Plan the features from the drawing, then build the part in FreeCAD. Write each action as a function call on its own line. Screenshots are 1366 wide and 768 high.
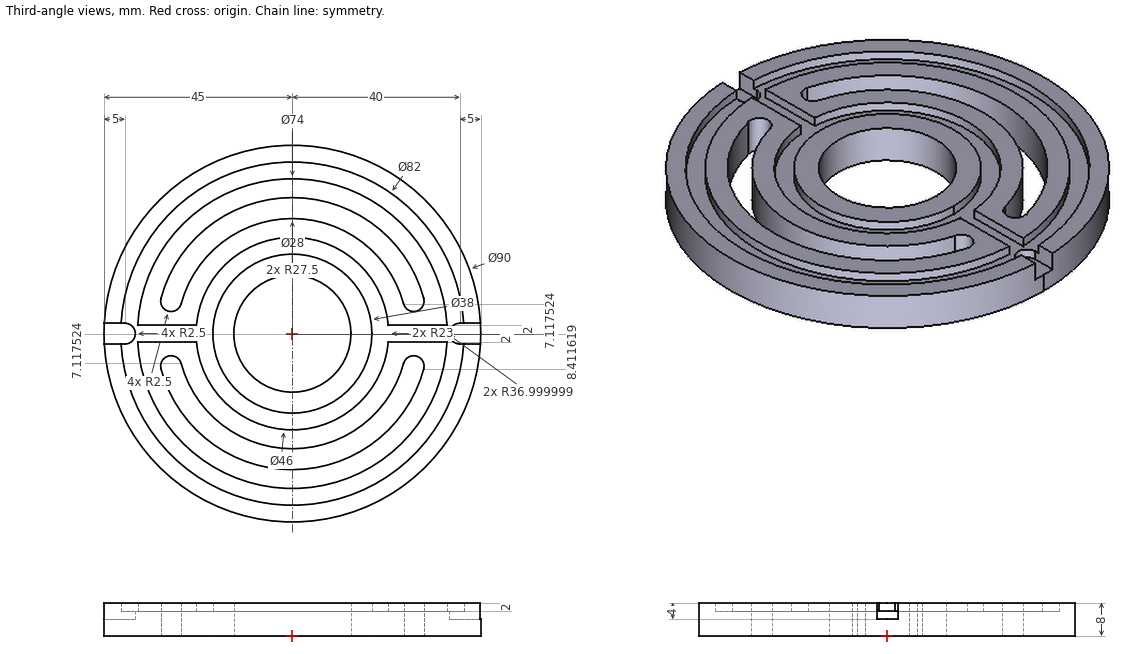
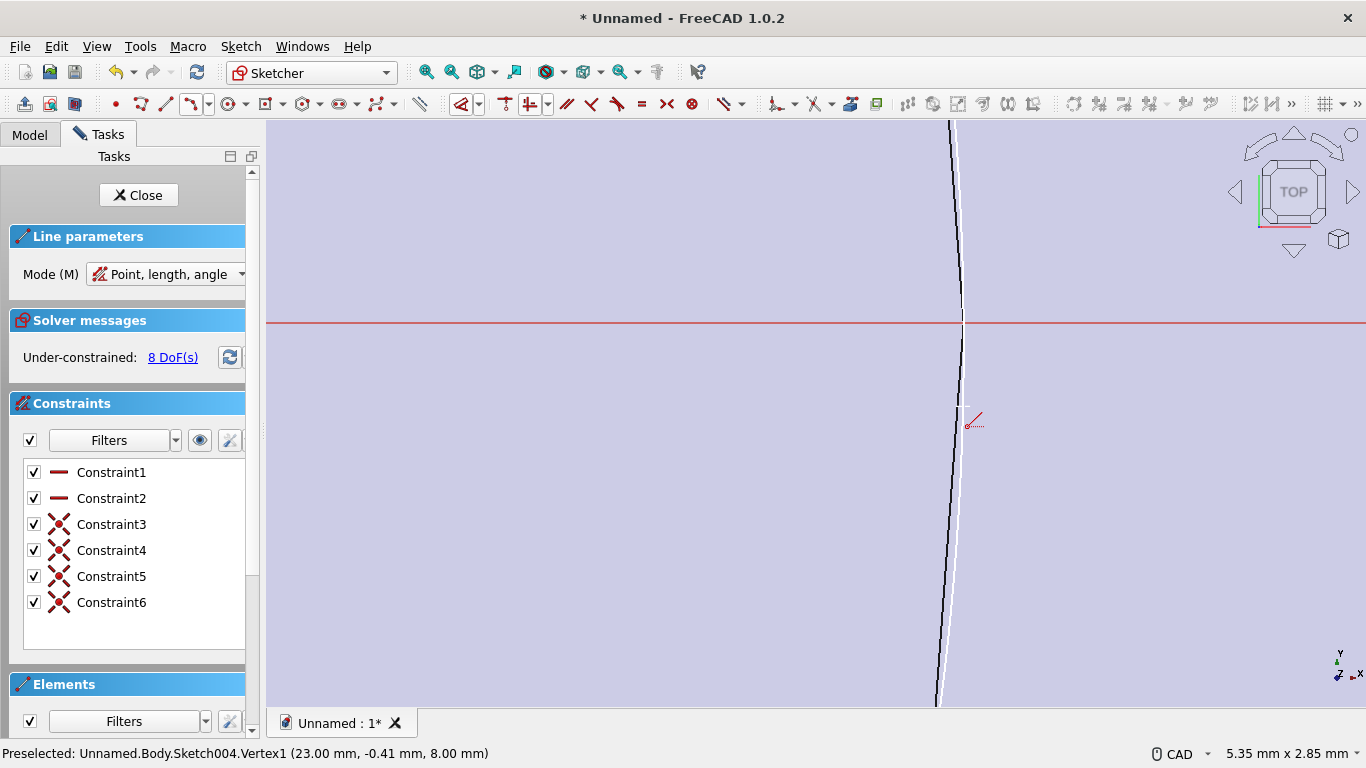
scroll(984, 418, down, 15)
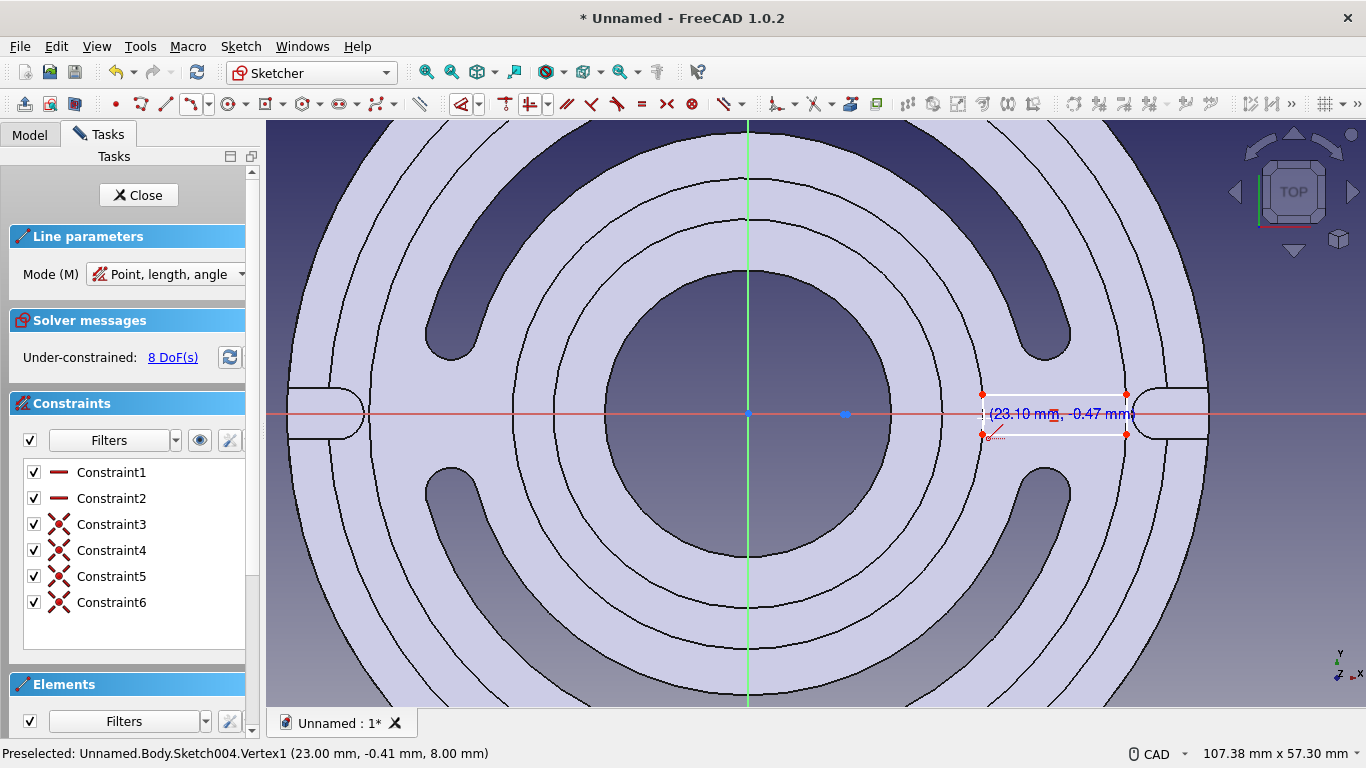
click(370, 434)
click(513, 434)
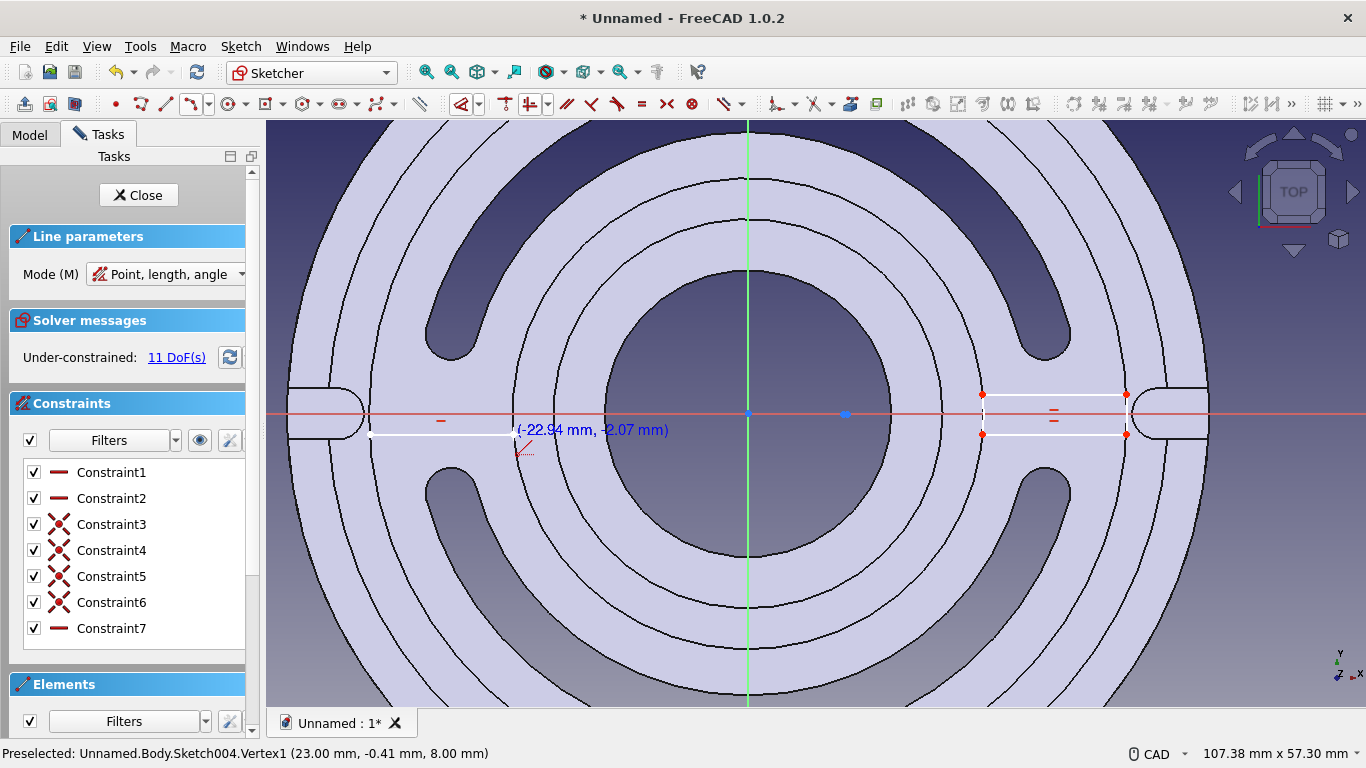
click(513, 393)
click(370, 393)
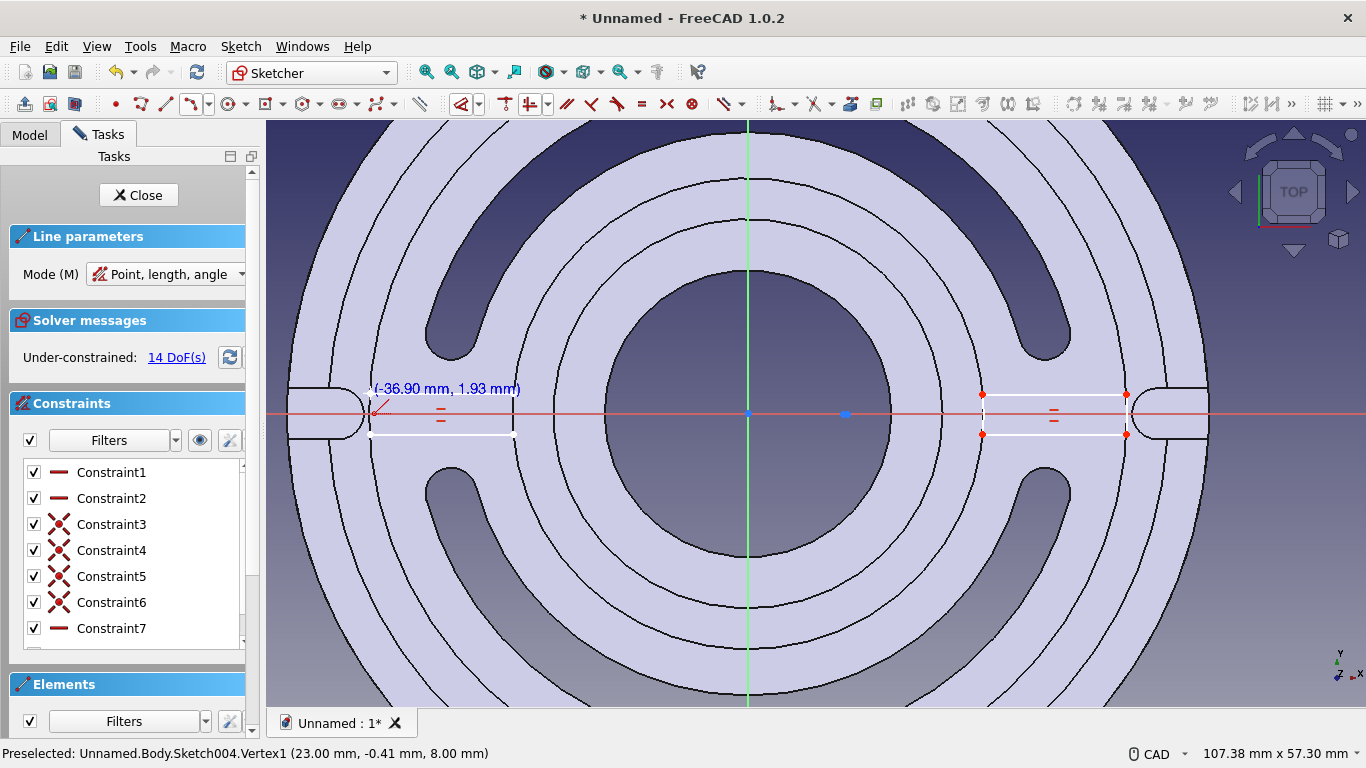
key(g)
key(3)
key(a)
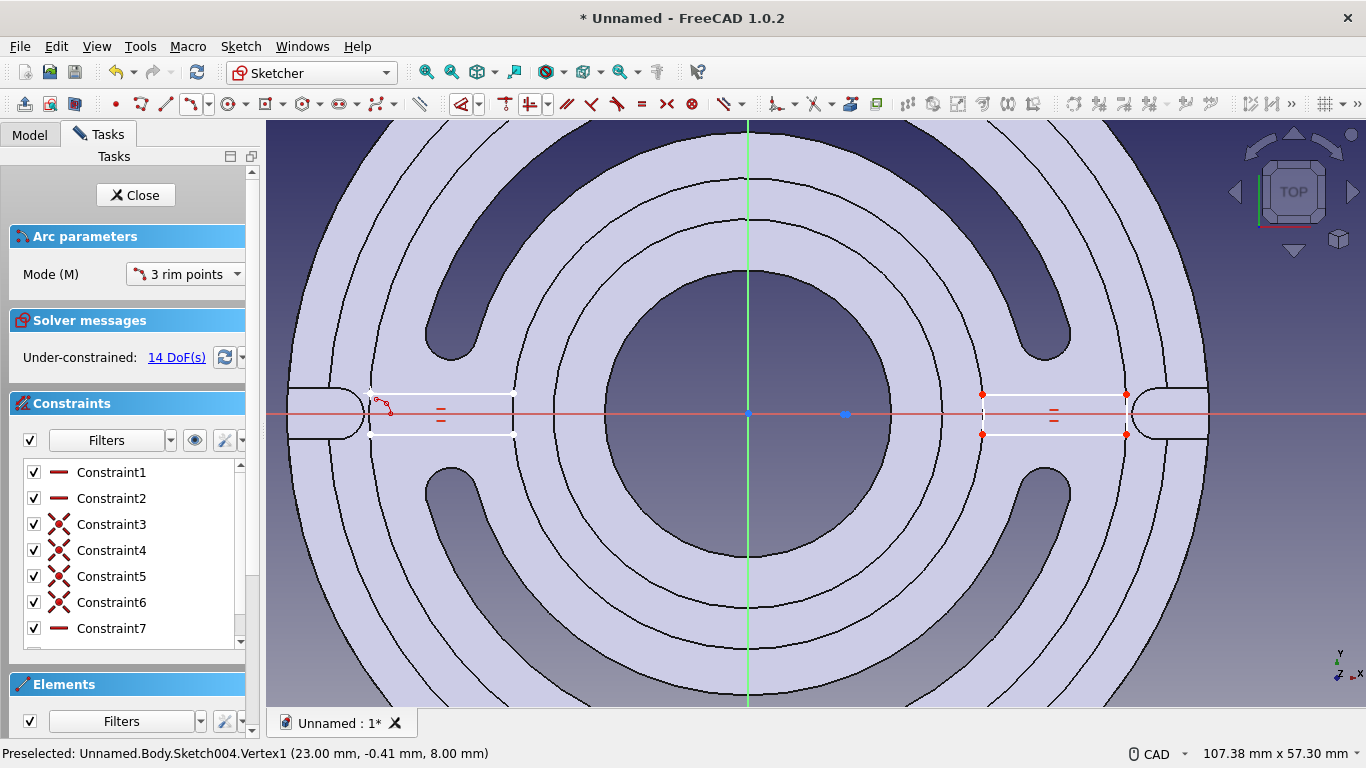
click(513, 435)
click(513, 394)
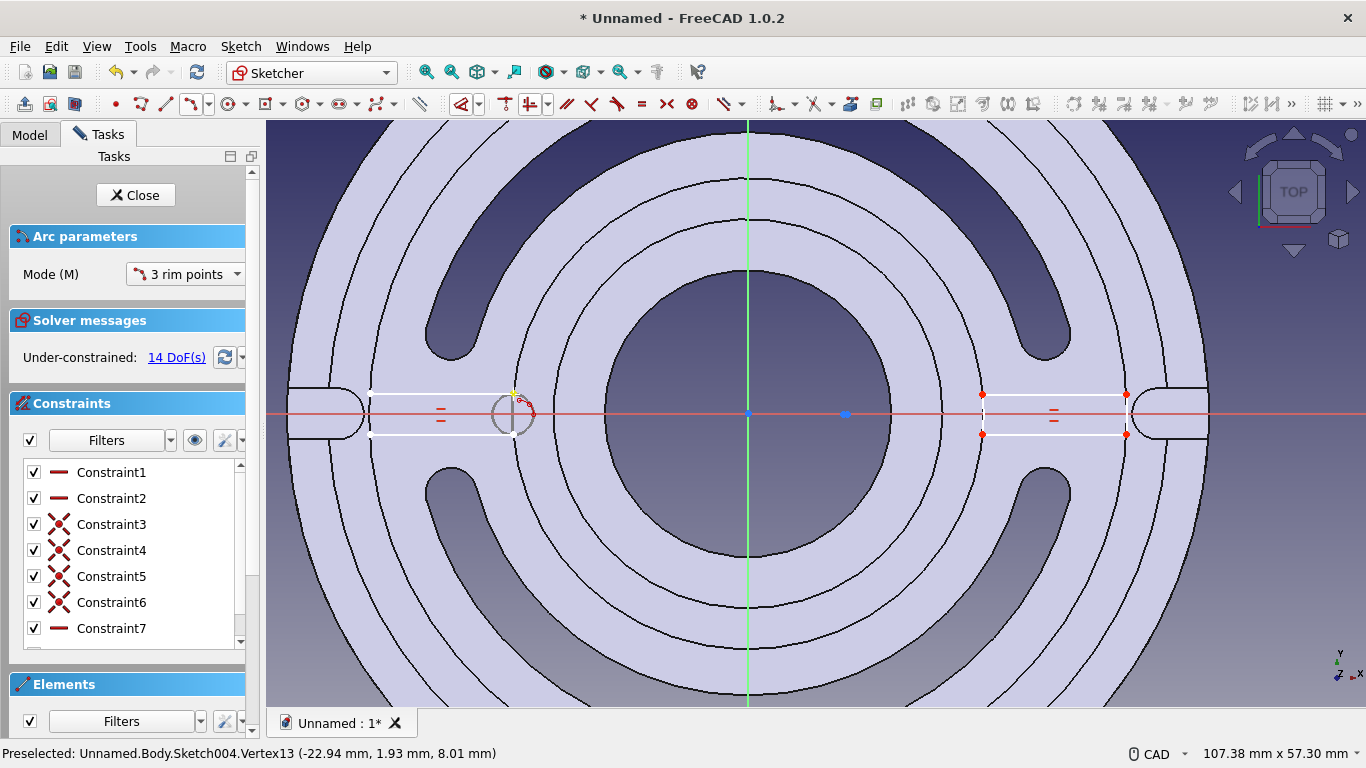
scroll(512, 410, up, 15)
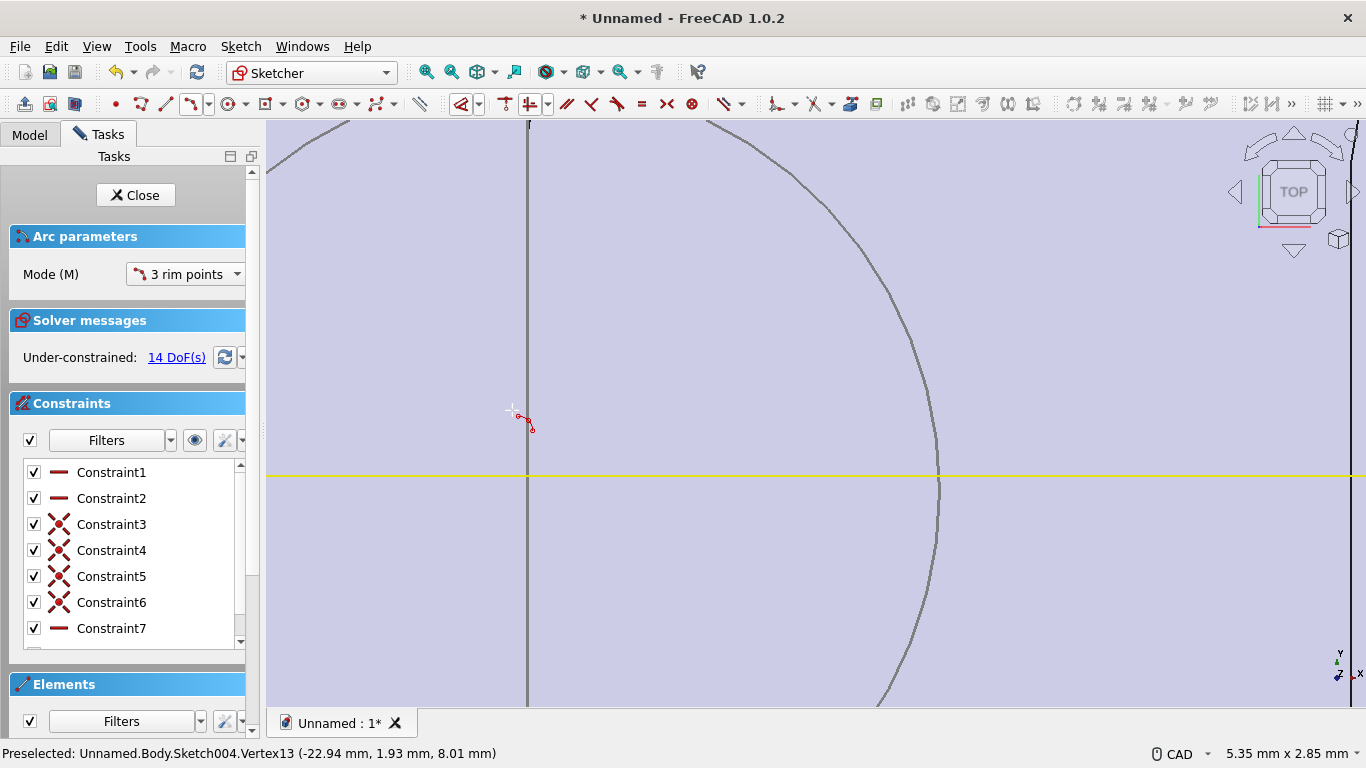
click(516, 394)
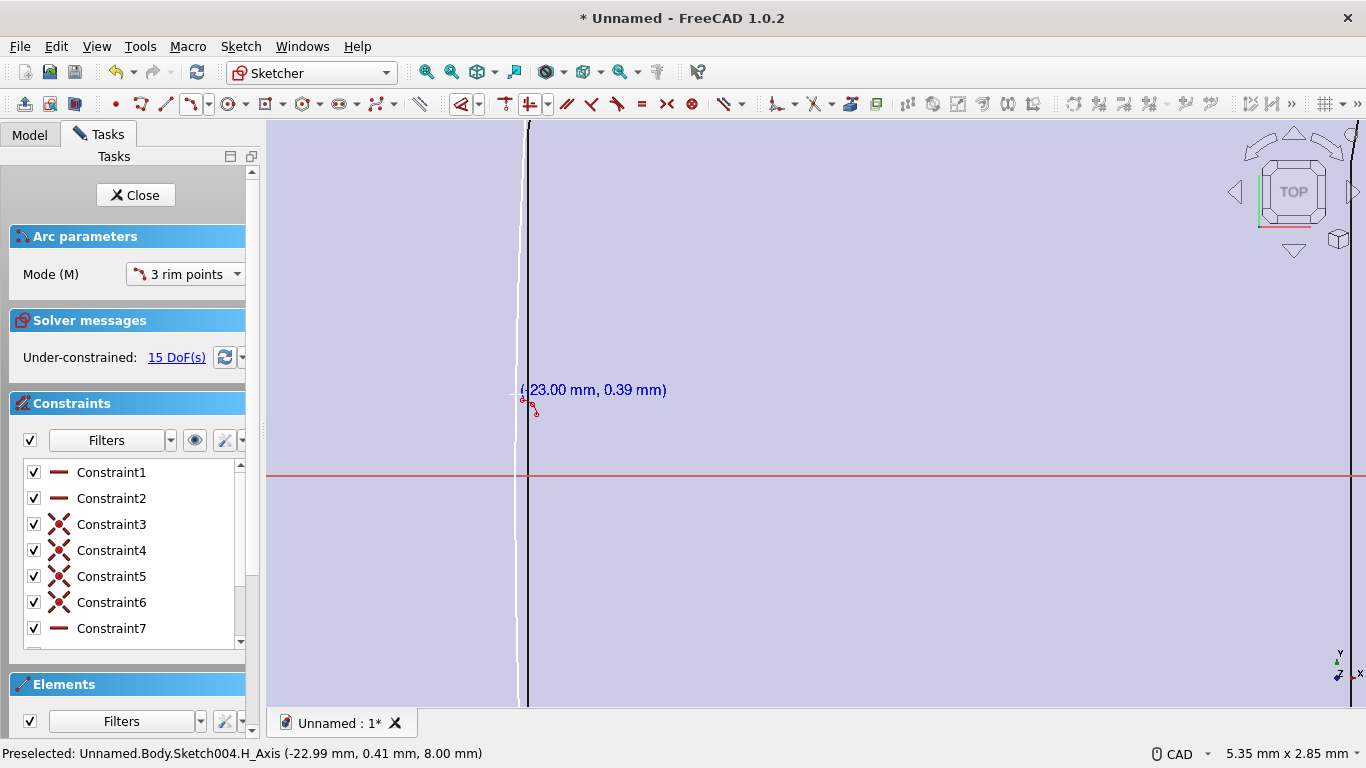
scroll(512, 410, down, 15)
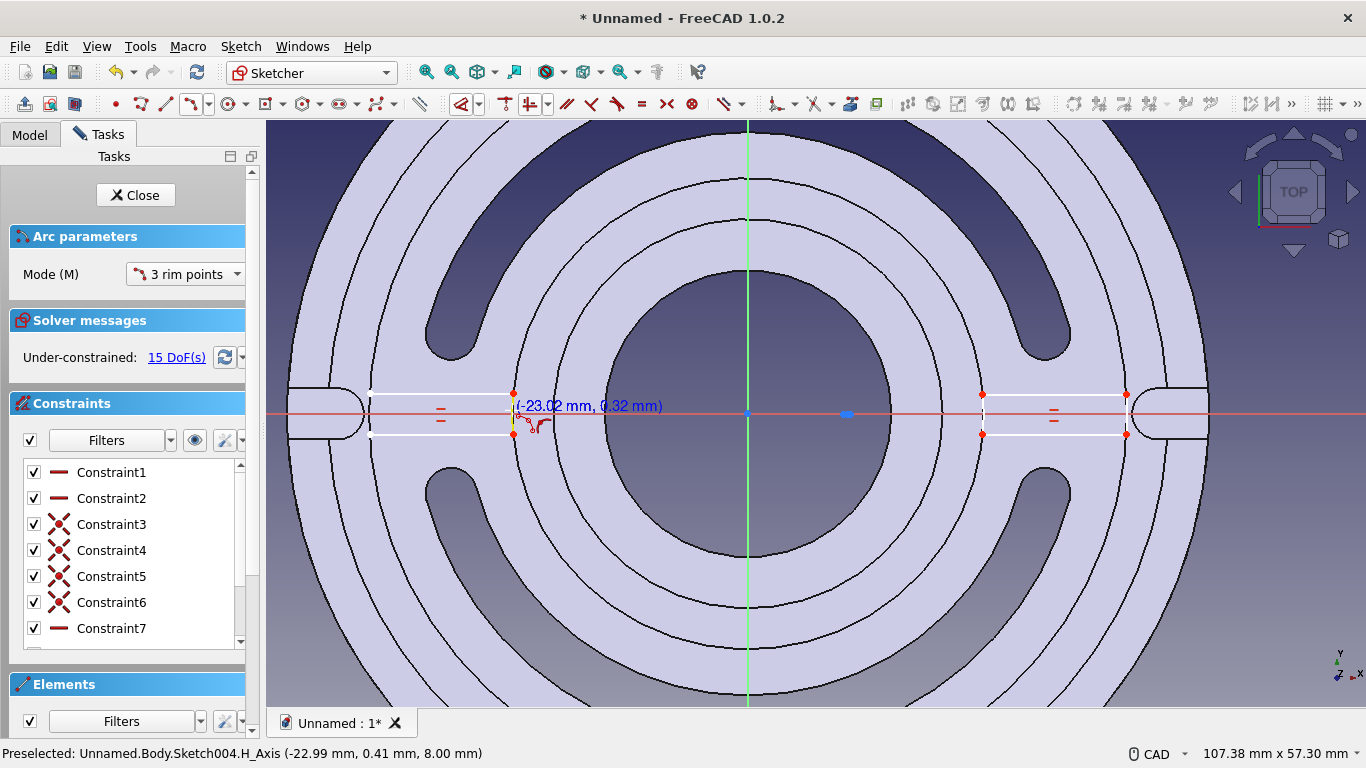
click(370, 394)
click(370, 435)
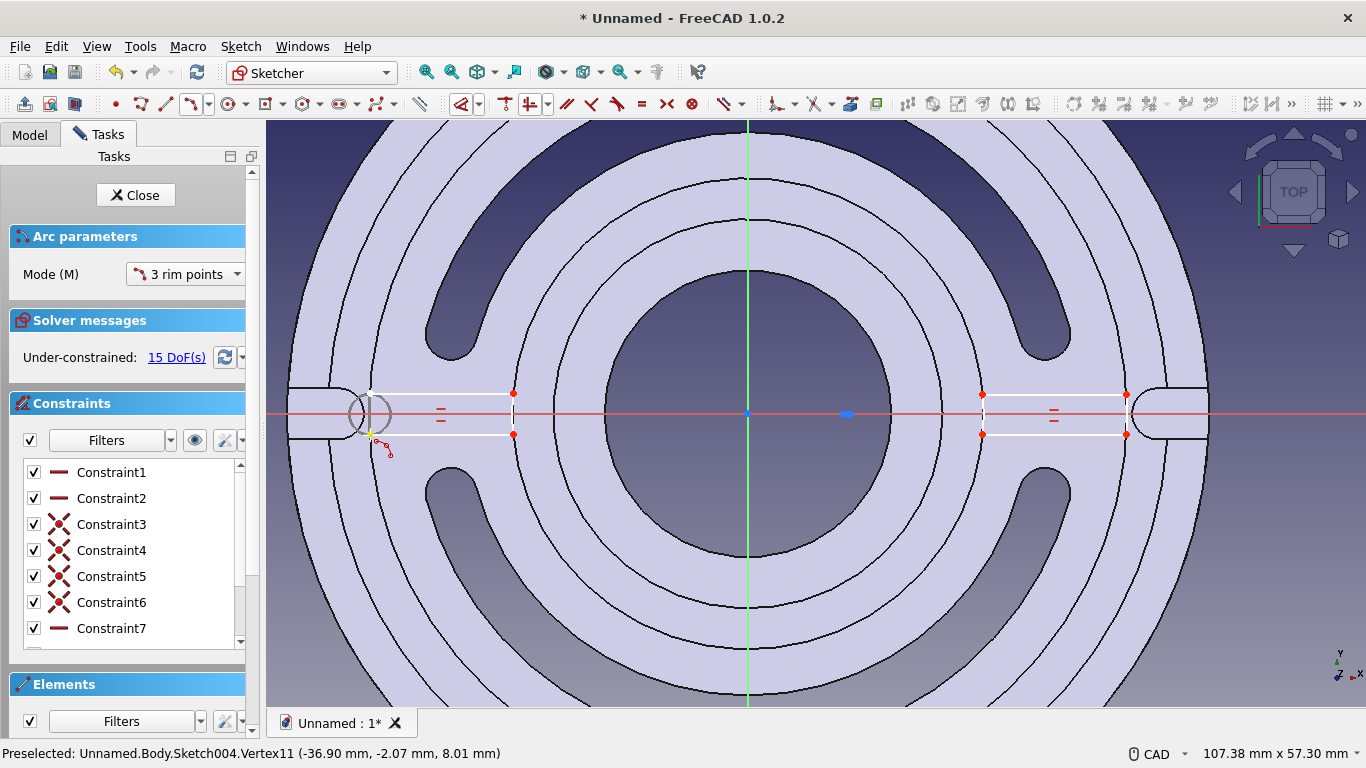
scroll(369, 410, up, 17)